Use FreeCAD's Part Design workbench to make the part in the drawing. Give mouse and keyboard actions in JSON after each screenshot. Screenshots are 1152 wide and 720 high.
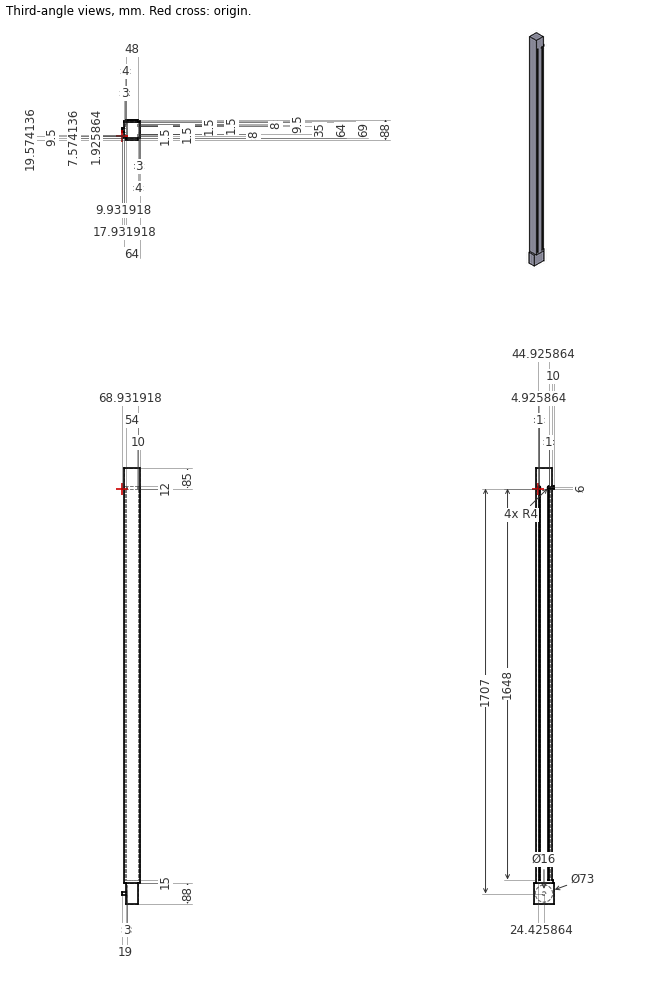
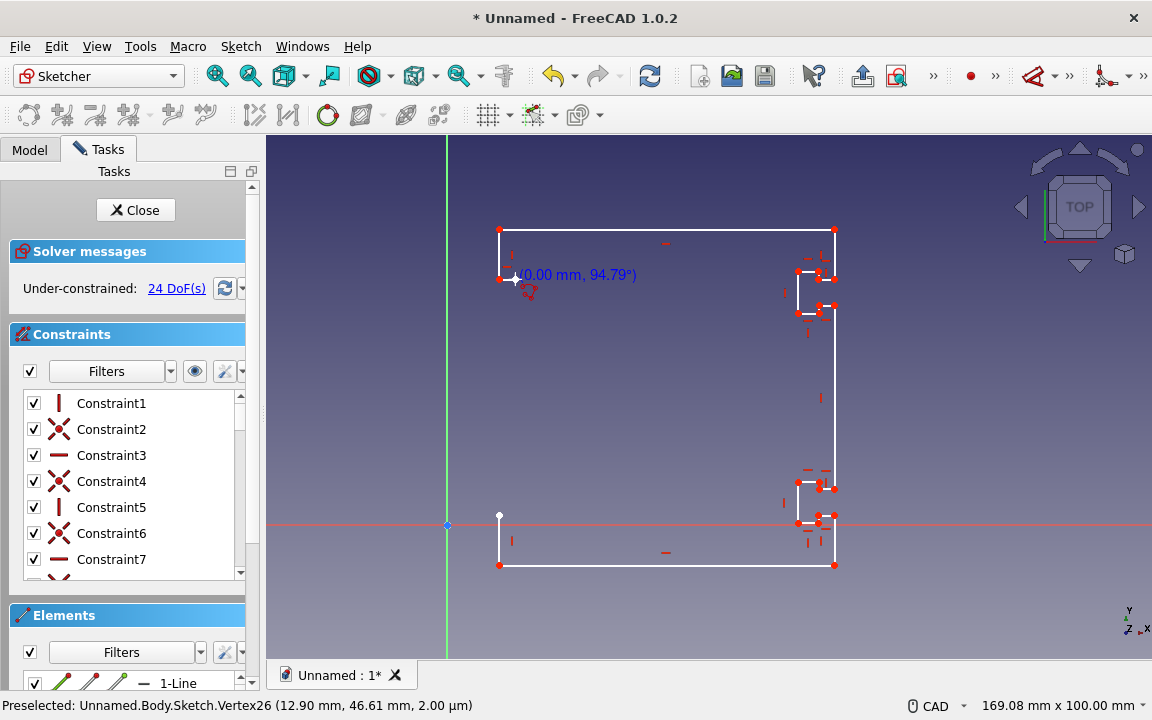
{"action": "scroll", "coordinate": [515, 271], "scroll_direction": "up", "scroll_amount": 4}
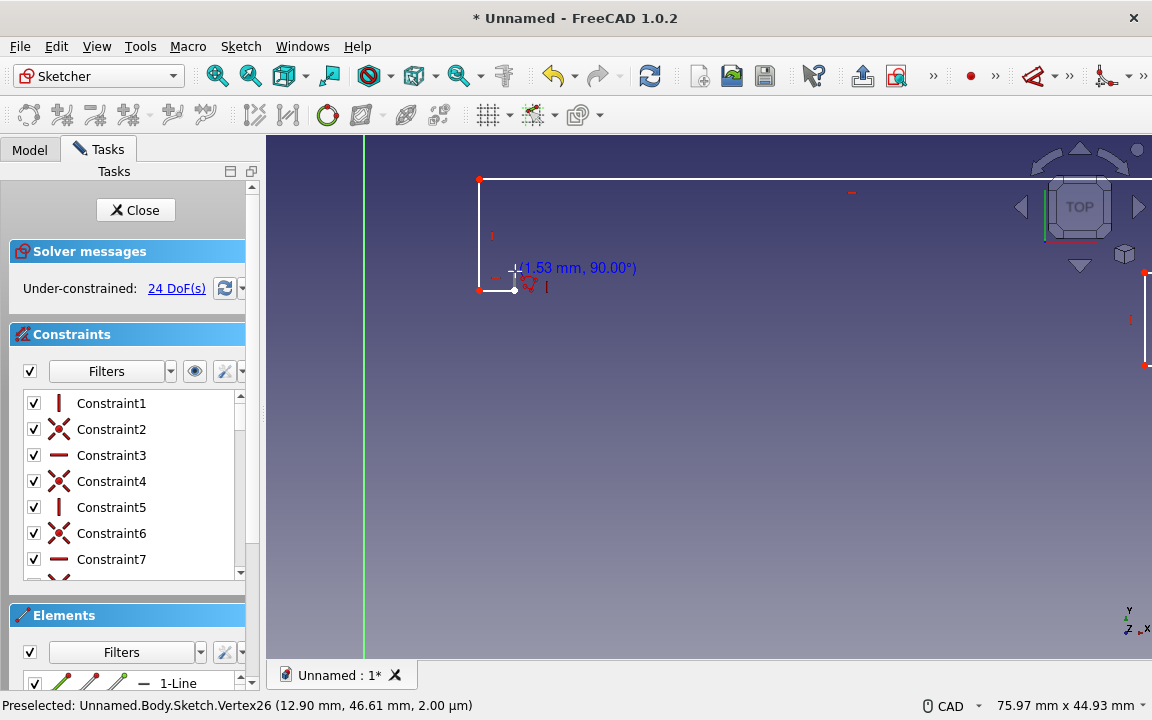
{"action": "left_click", "coordinate": [515, 272]}
{"action": "left_click", "coordinate": [562, 272]}
{"action": "left_click", "coordinate": [562, 365]}
{"action": "left_click", "coordinate": [515, 365]}
{"action": "left_click", "coordinate": [515, 347]}
{"action": "left_click", "coordinate": [480, 347]}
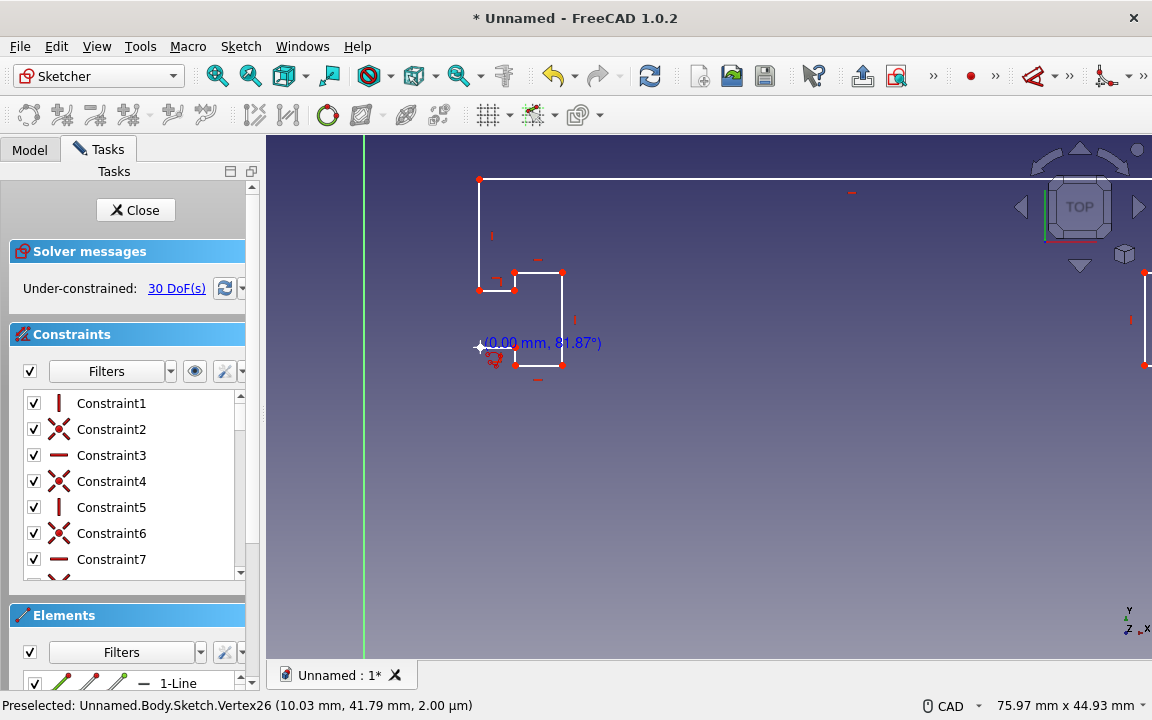
{"action": "scroll", "coordinate": [514, 271], "scroll_direction": "down", "scroll_amount": 4}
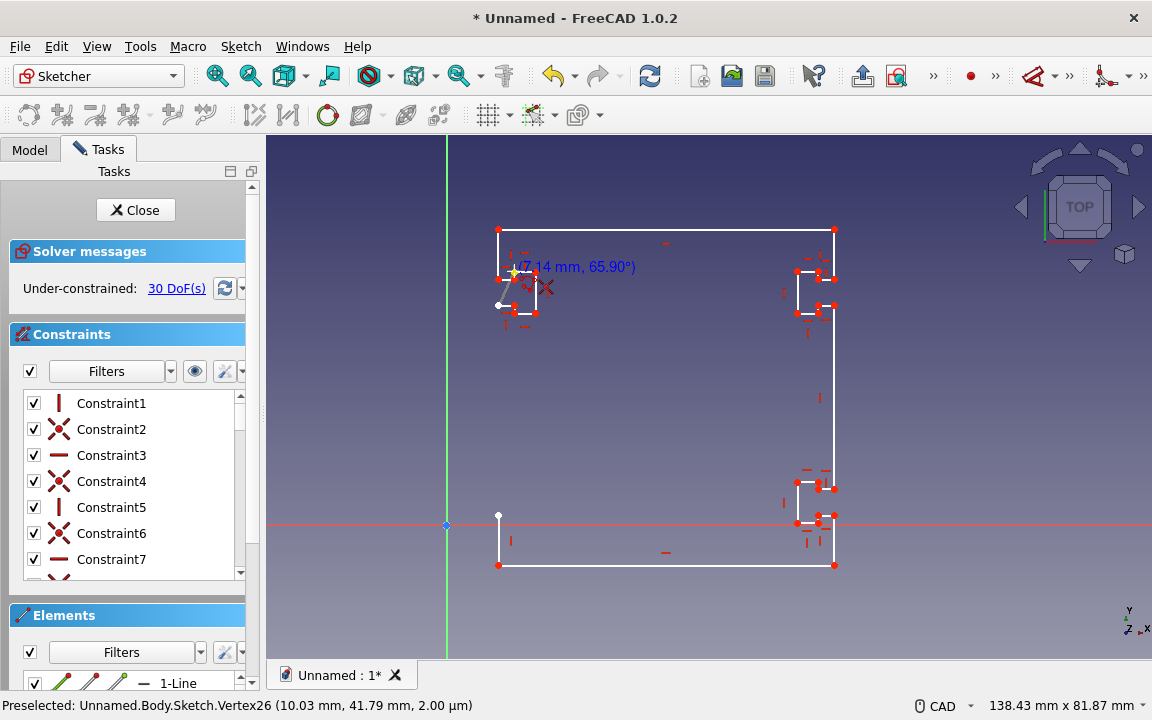
{"action": "left_click", "coordinate": [499, 489]}
{"action": "left_click", "coordinate": [515, 489]}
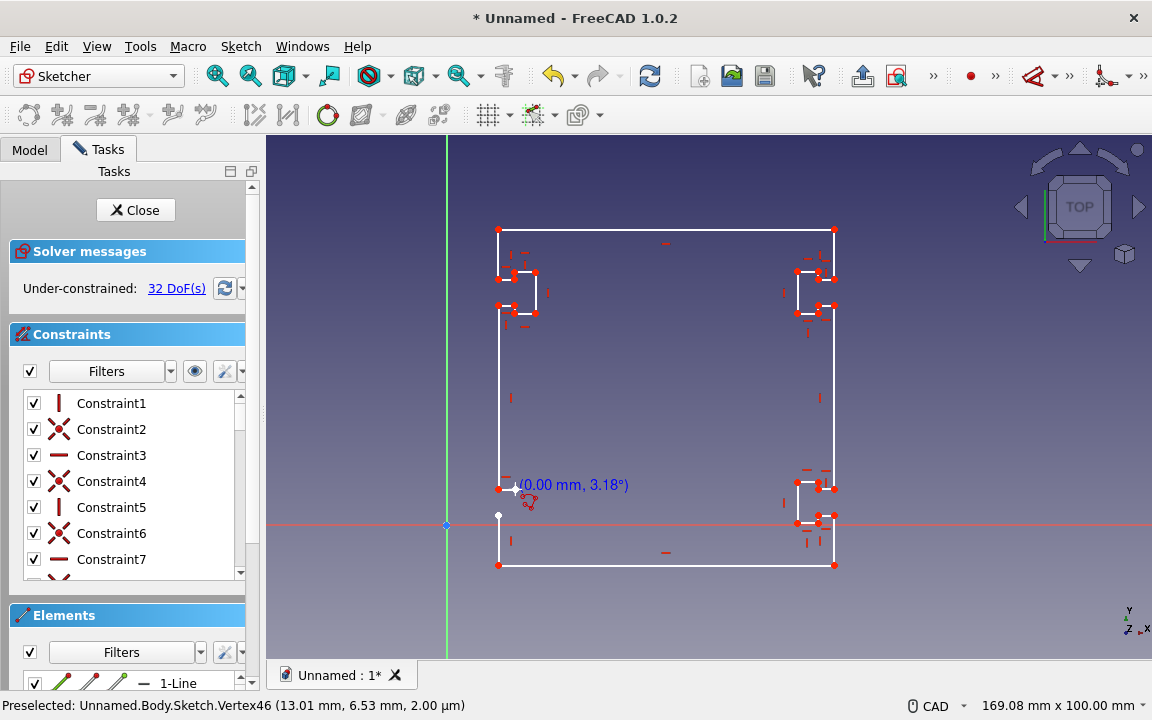
{"action": "scroll", "coordinate": [515, 481], "scroll_direction": "up", "scroll_amount": 4}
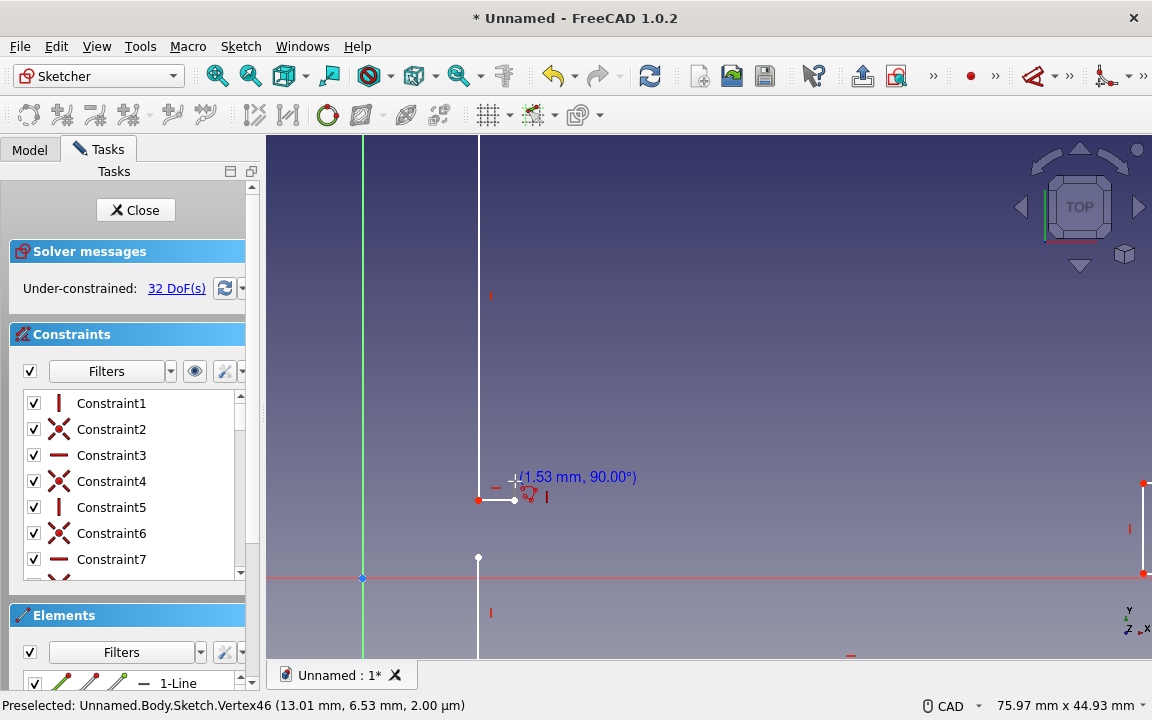
{"action": "left_click", "coordinate": [515, 480]}
{"action": "left_click", "coordinate": [560, 480]}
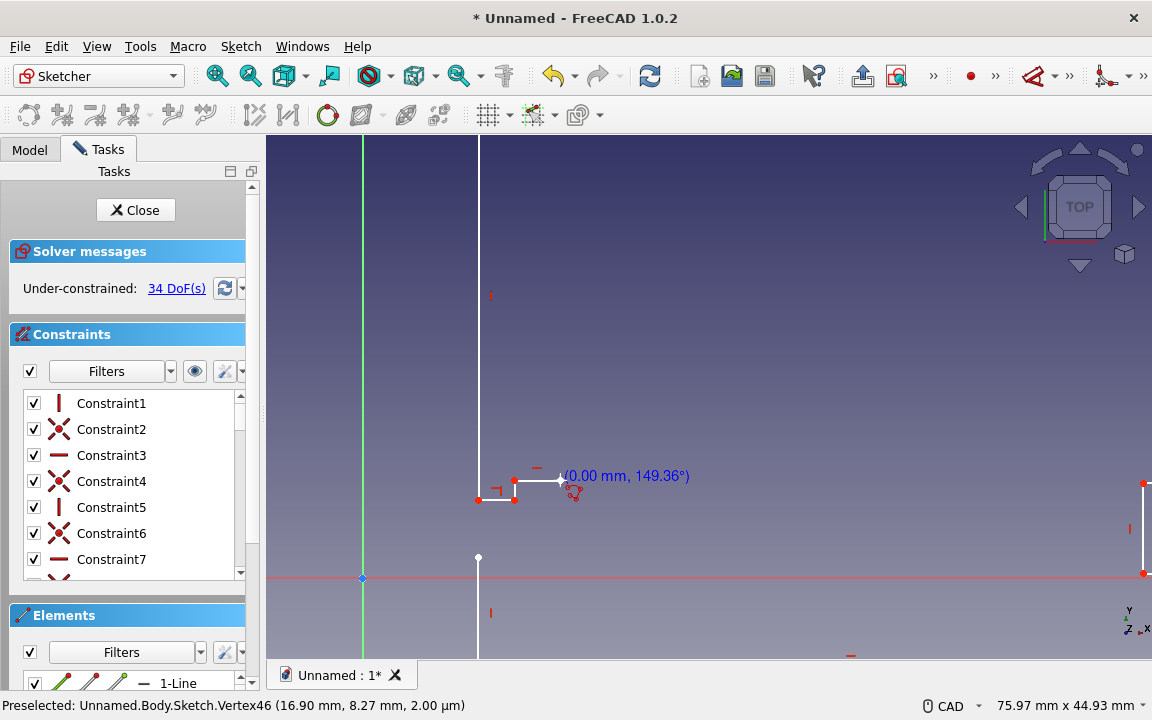
{"action": "scroll", "coordinate": [560, 574], "scroll_direction": "up", "scroll_amount": 6}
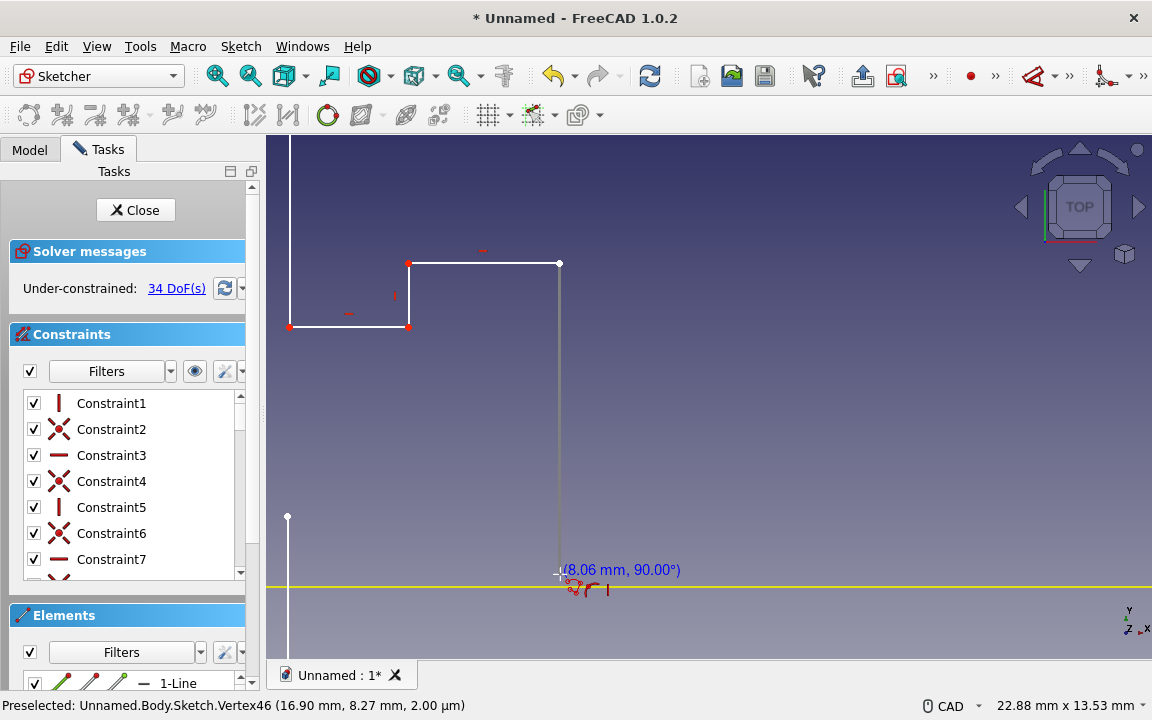
{"action": "left_click", "coordinate": [559, 570]}
{"action": "left_click", "coordinate": [405, 570]}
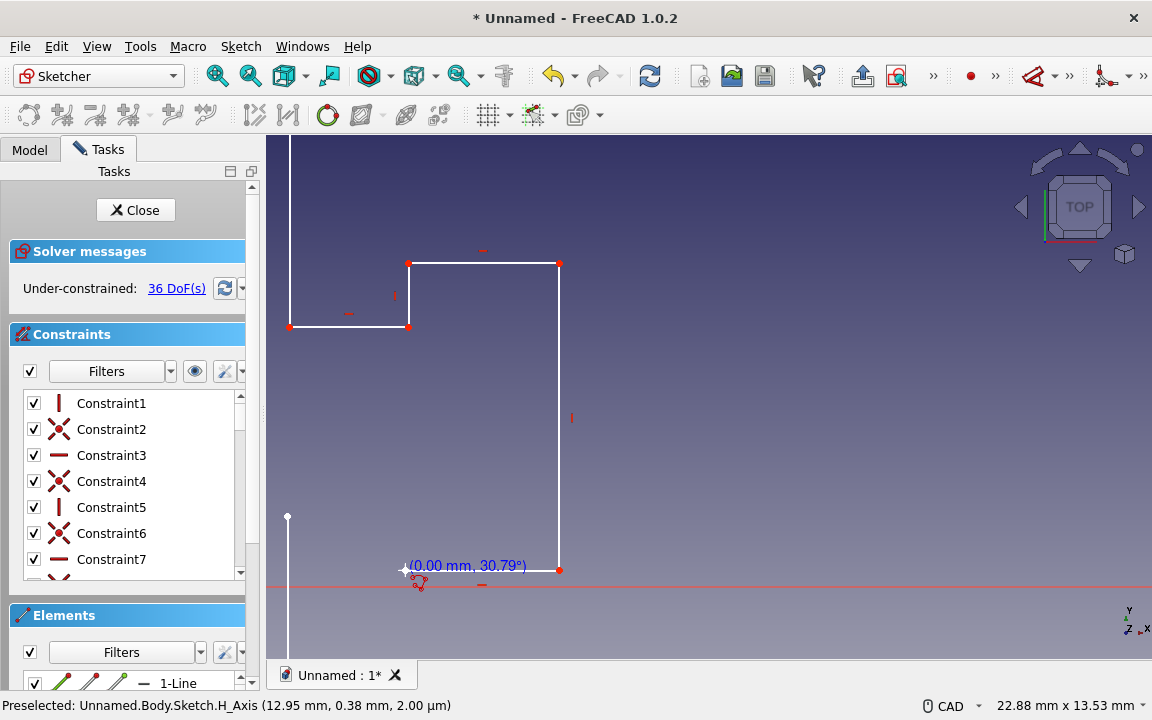
{"action": "scroll", "coordinate": [532, 515], "scroll_direction": "down", "scroll_amount": 10}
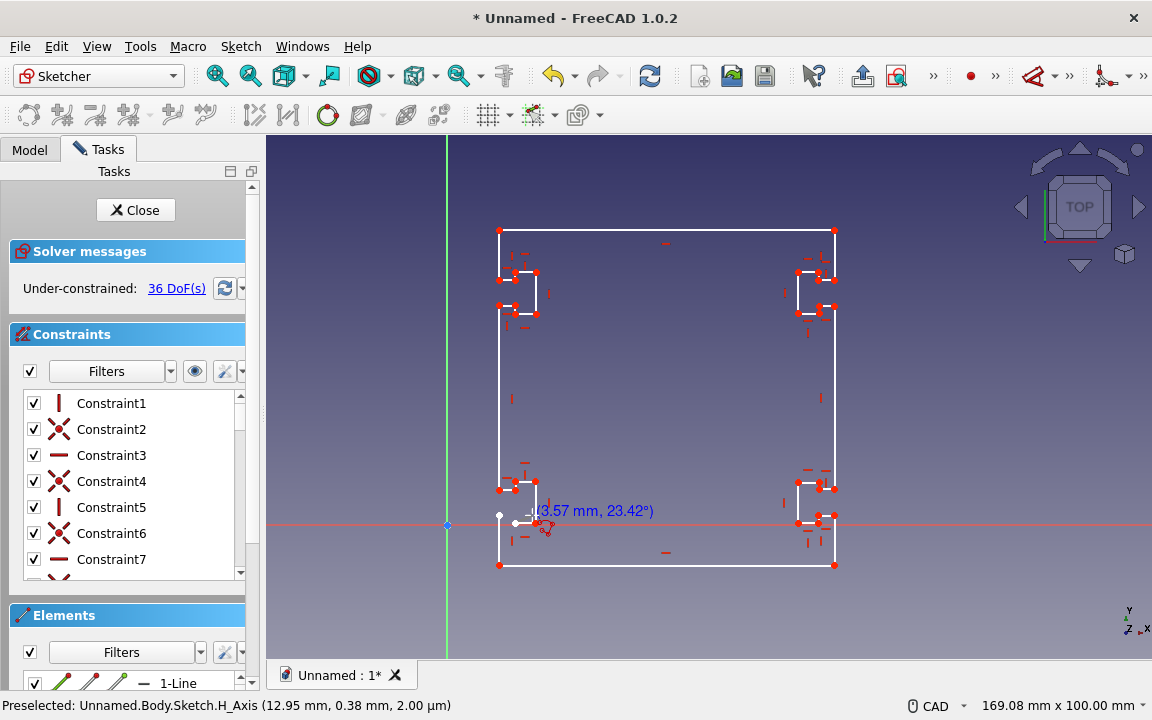
{"action": "scroll", "coordinate": [515, 515], "scroll_direction": "up", "scroll_amount": 4}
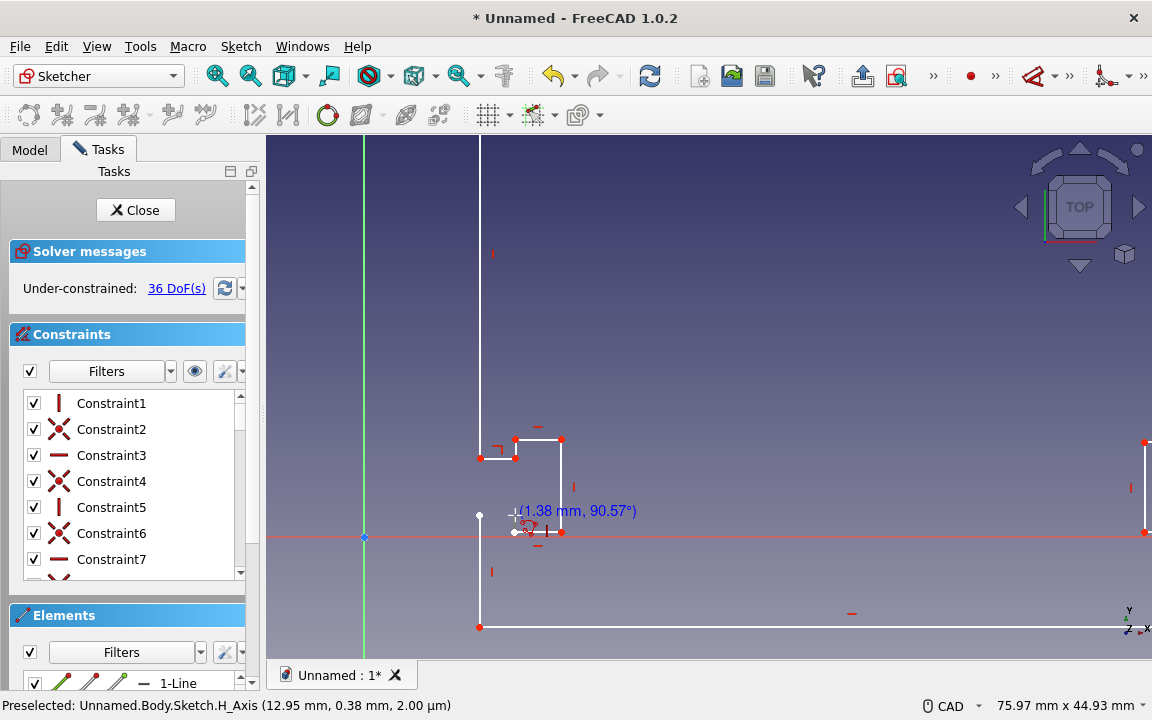
{"action": "left_click", "coordinate": [515, 515]}
{"action": "left_click", "coordinate": [480, 516]}
{"action": "key", "text": "Escape"}
{"action": "key", "text": "Escape"}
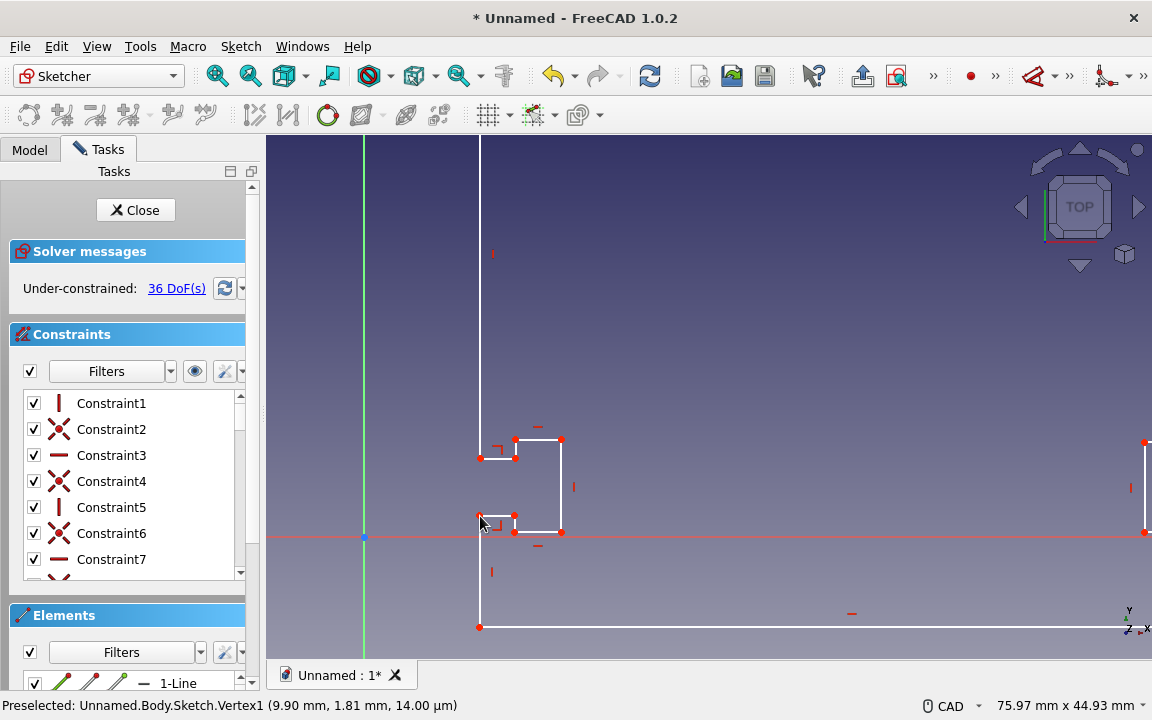
{"action": "left_click", "coordinate": [1032, 76]}